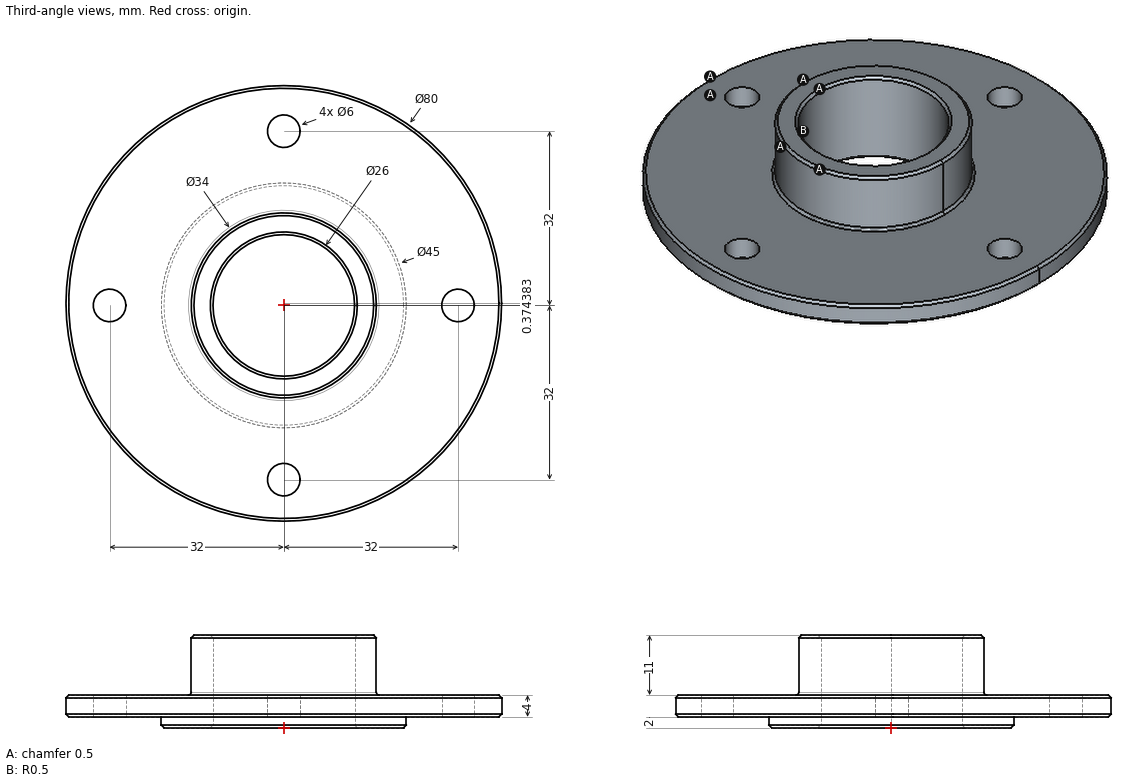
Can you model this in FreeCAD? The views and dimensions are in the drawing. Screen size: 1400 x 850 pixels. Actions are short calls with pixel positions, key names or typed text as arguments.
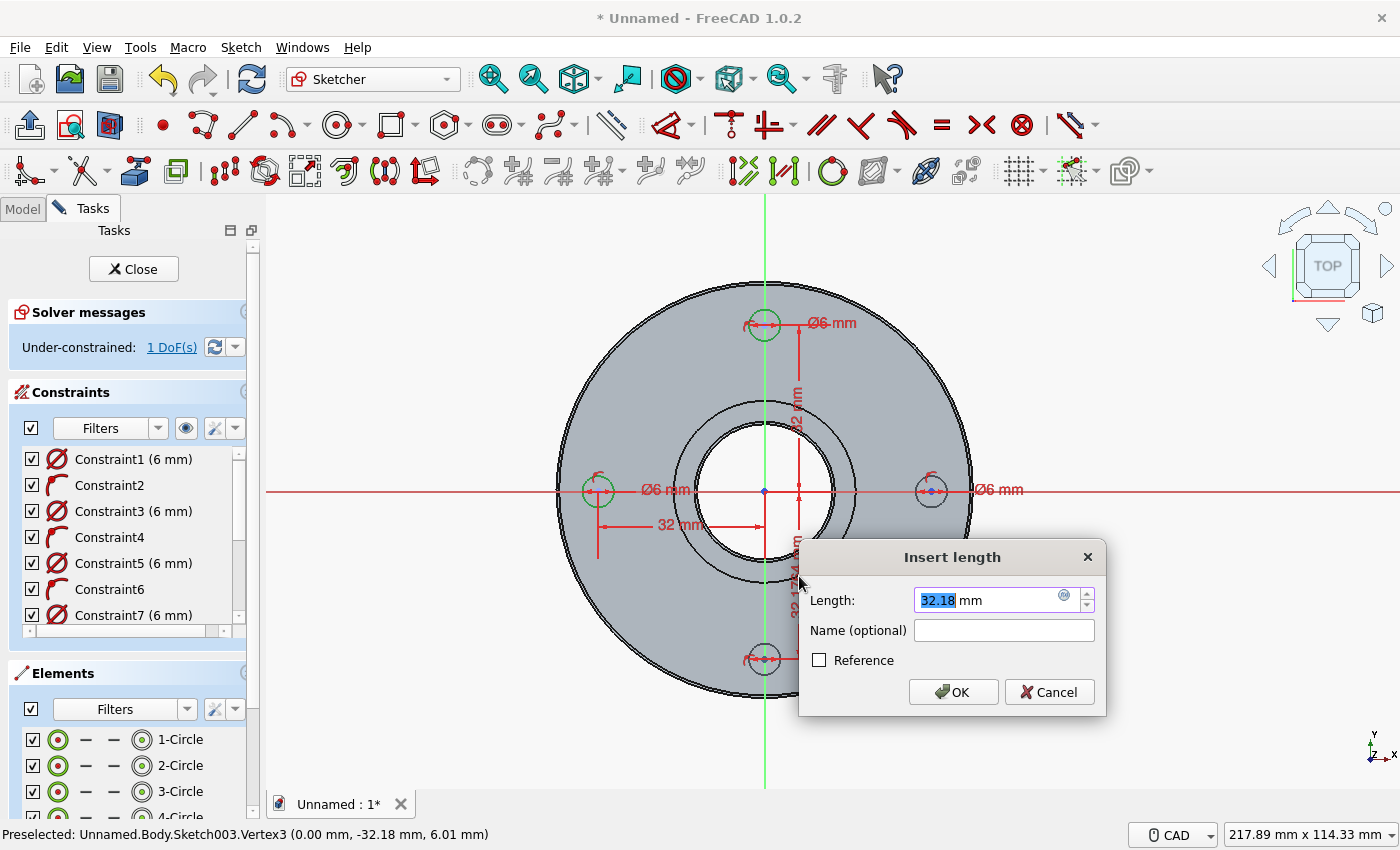
text(32)
key(Return)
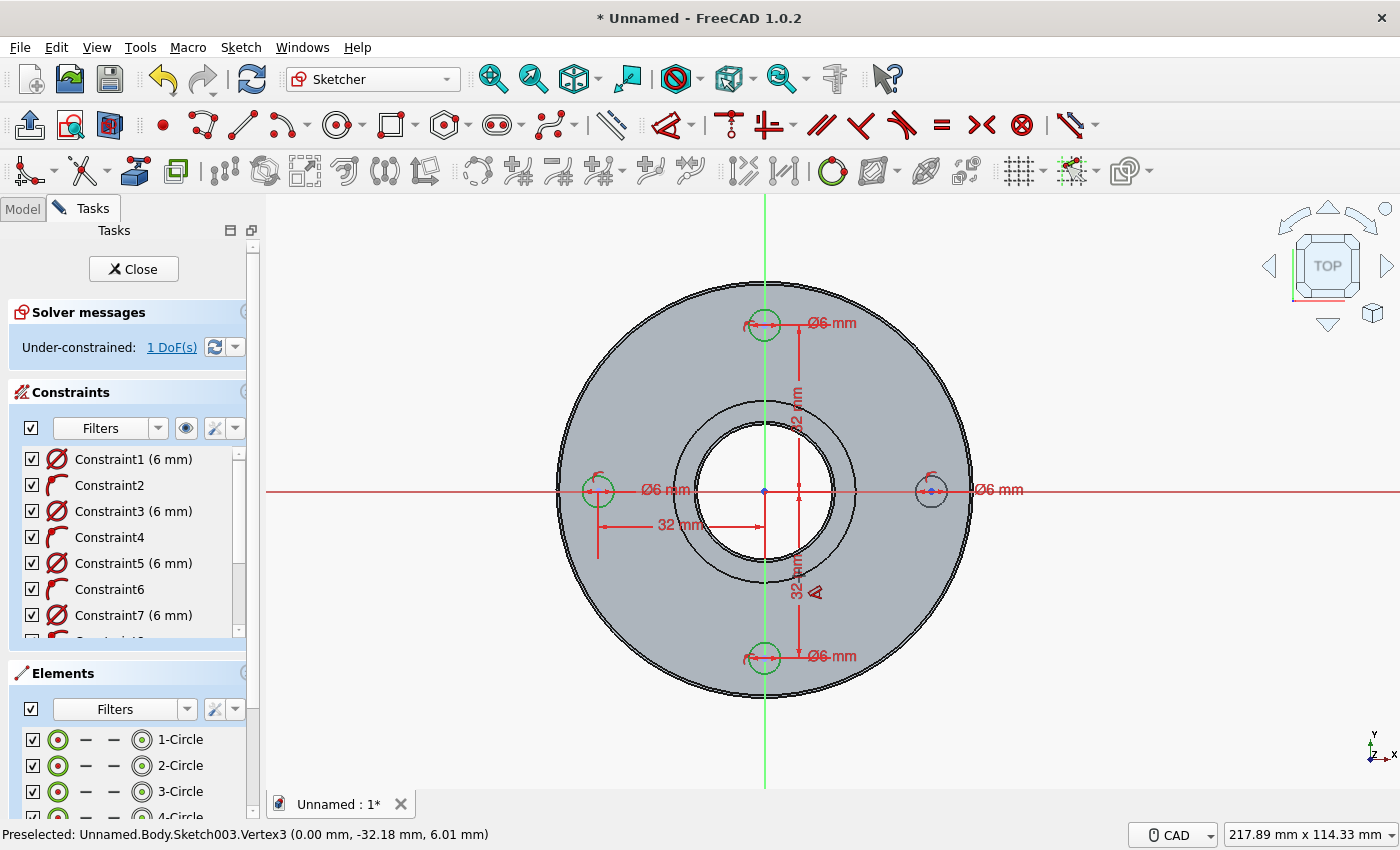
click(931, 492)
click(848, 526)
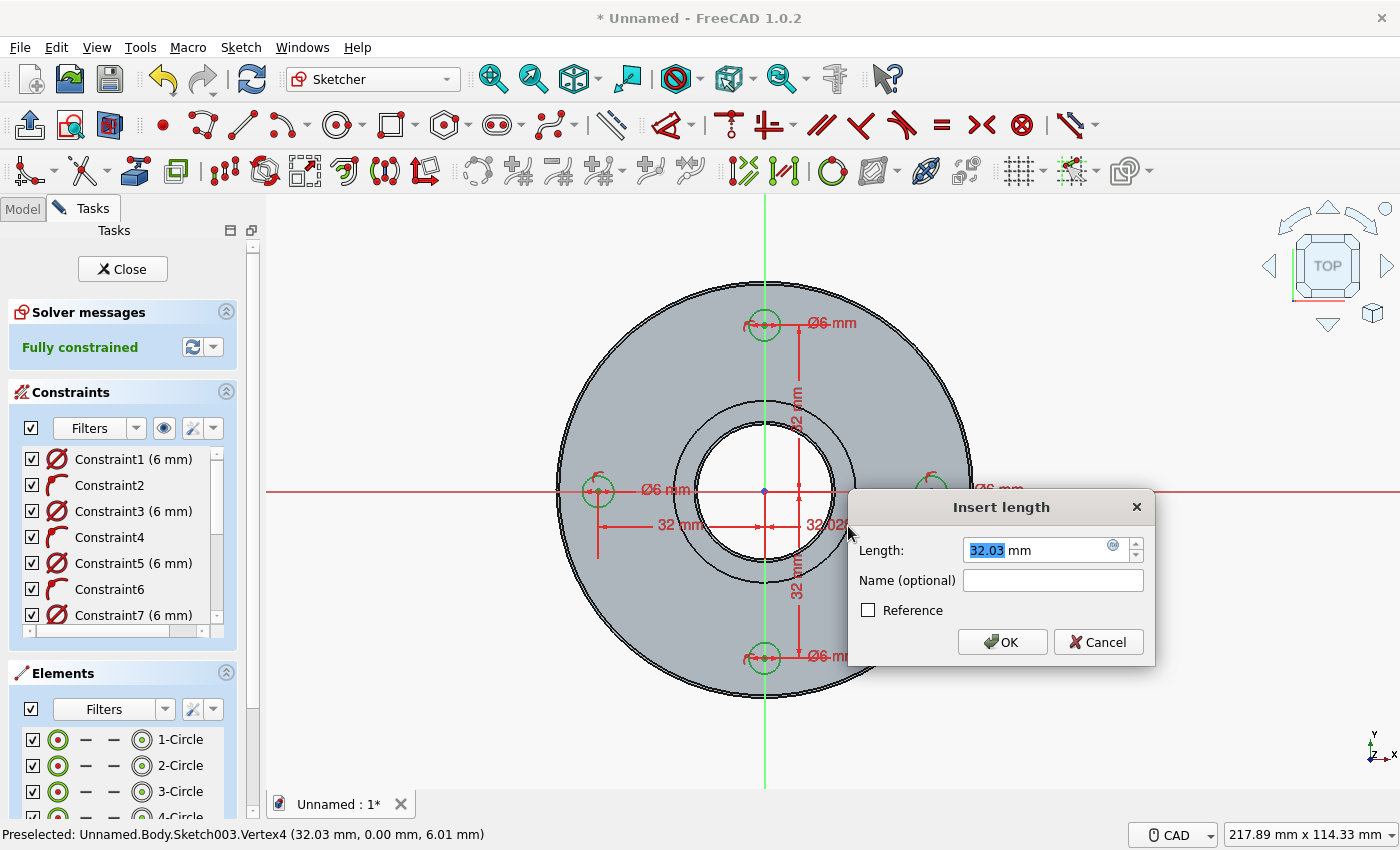
text(32)
key(Return)
key(Escape)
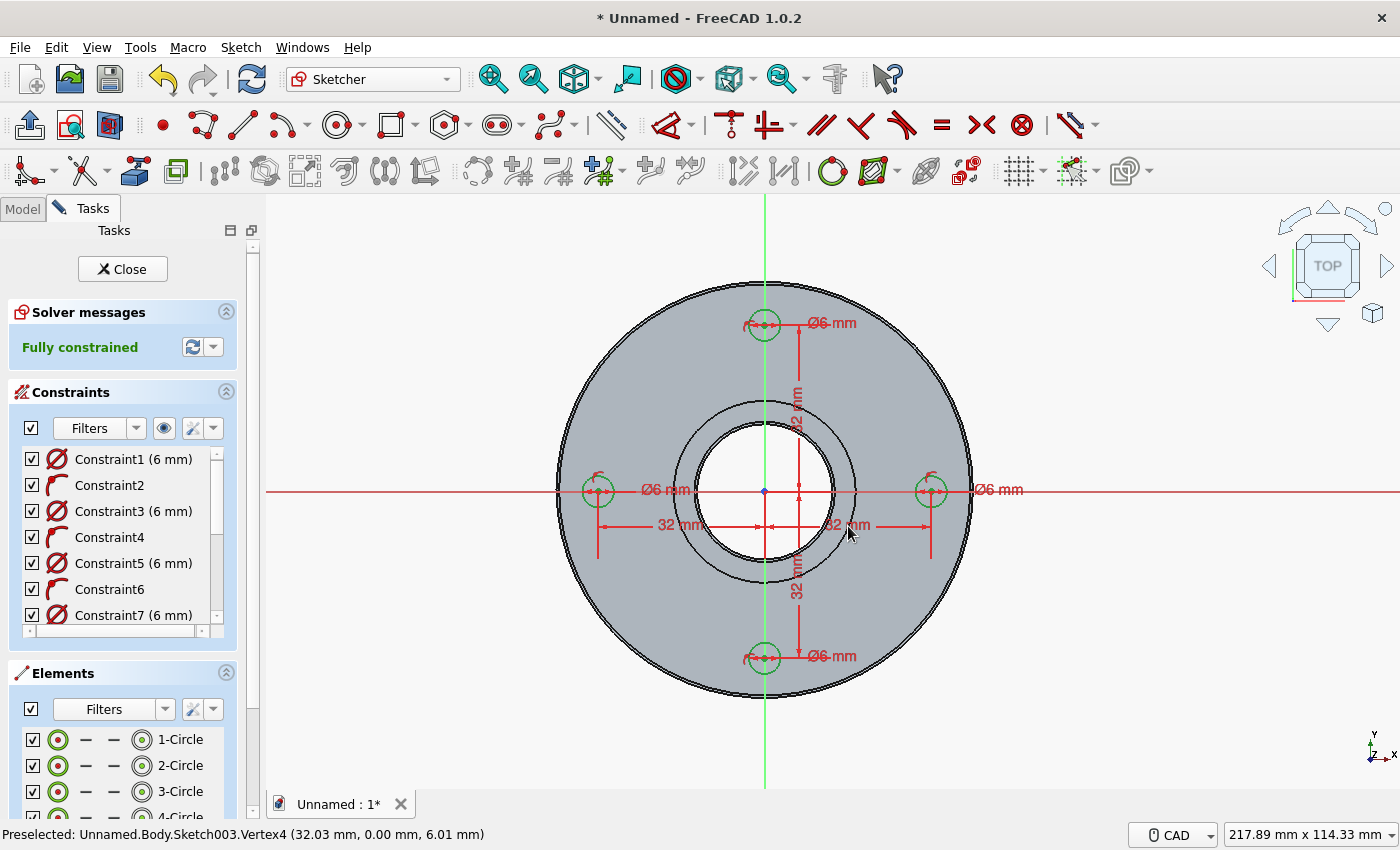
click(123, 269)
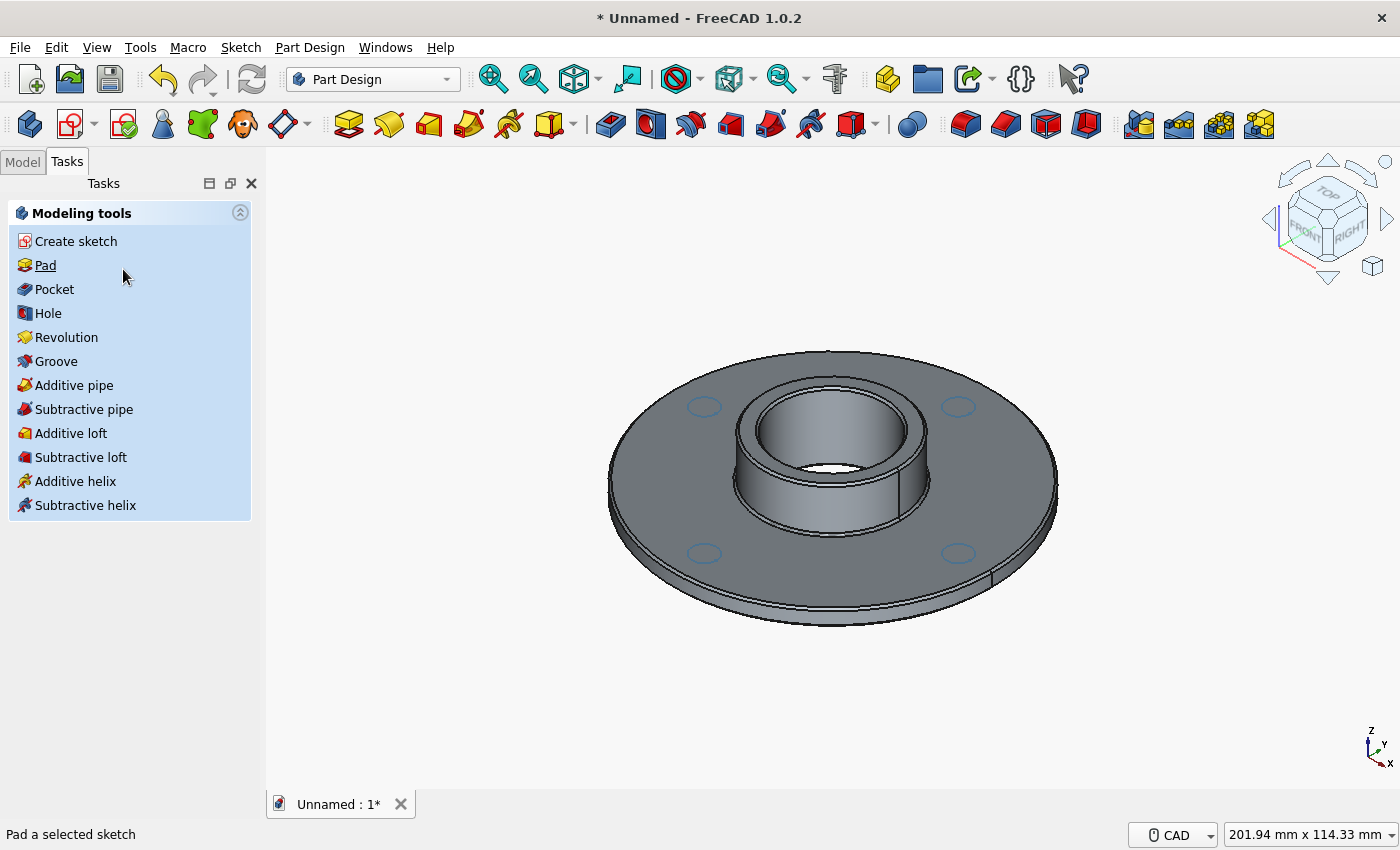
click(612, 124)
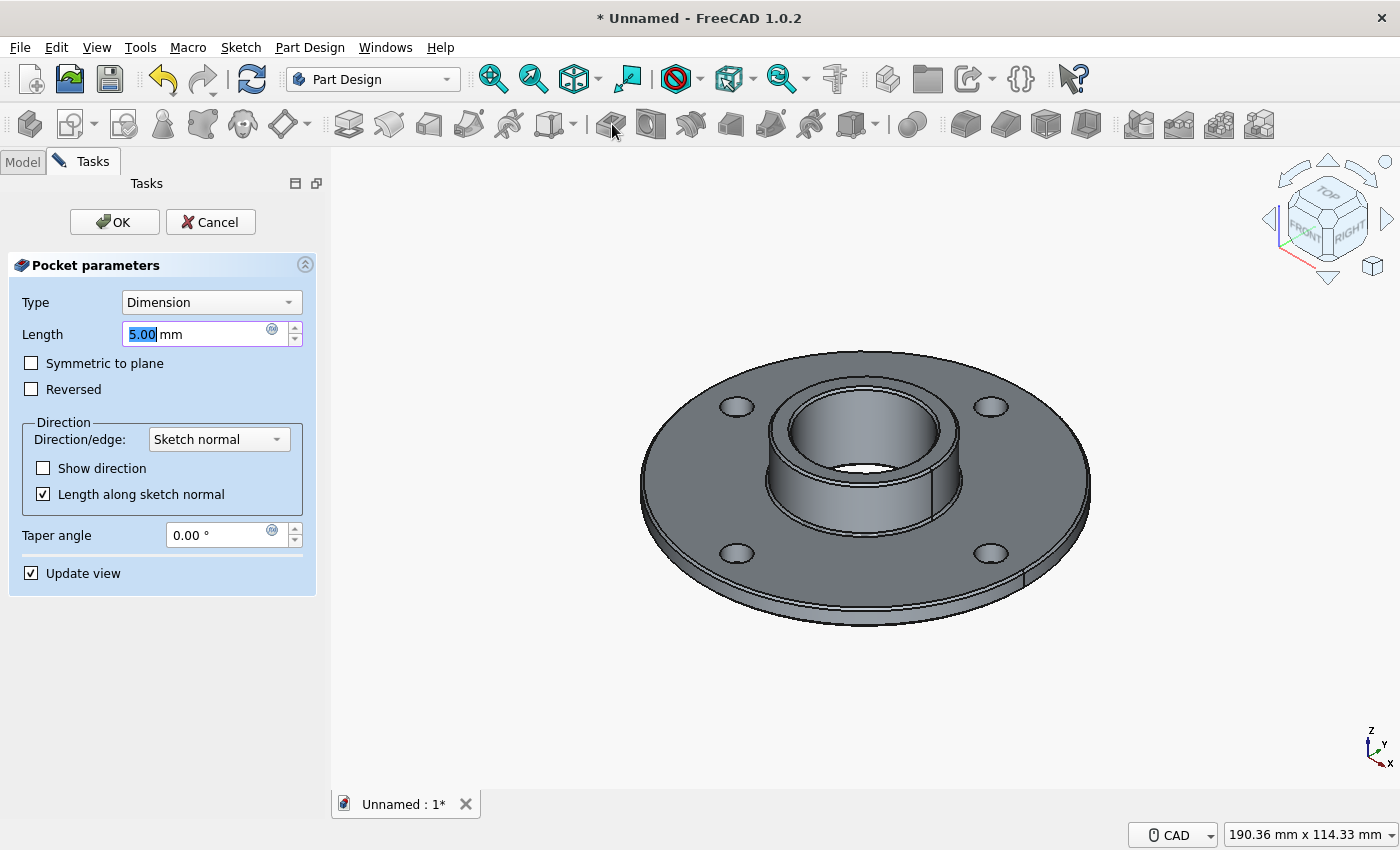
click(212, 302)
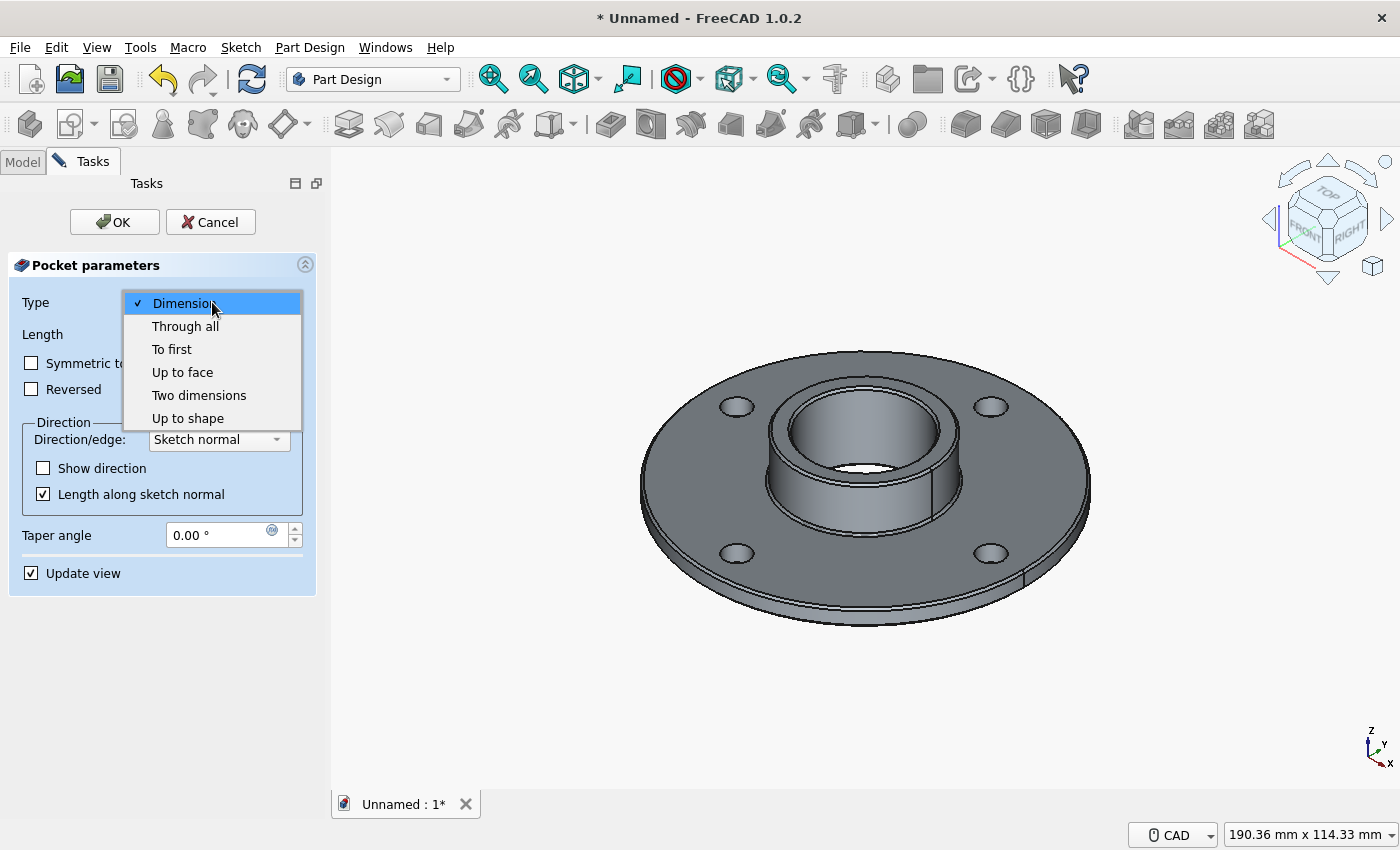
click(212, 326)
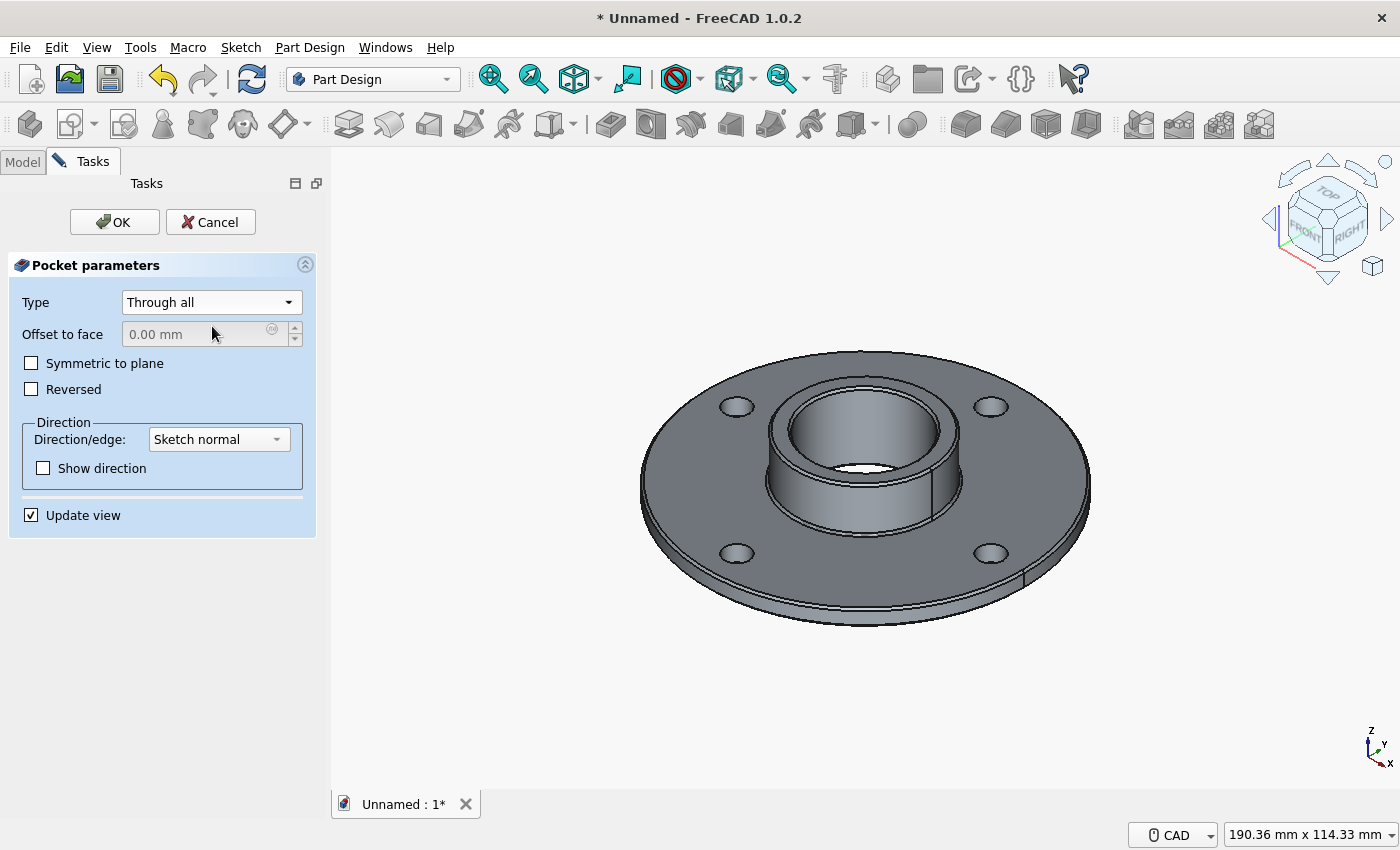
click(115, 222)